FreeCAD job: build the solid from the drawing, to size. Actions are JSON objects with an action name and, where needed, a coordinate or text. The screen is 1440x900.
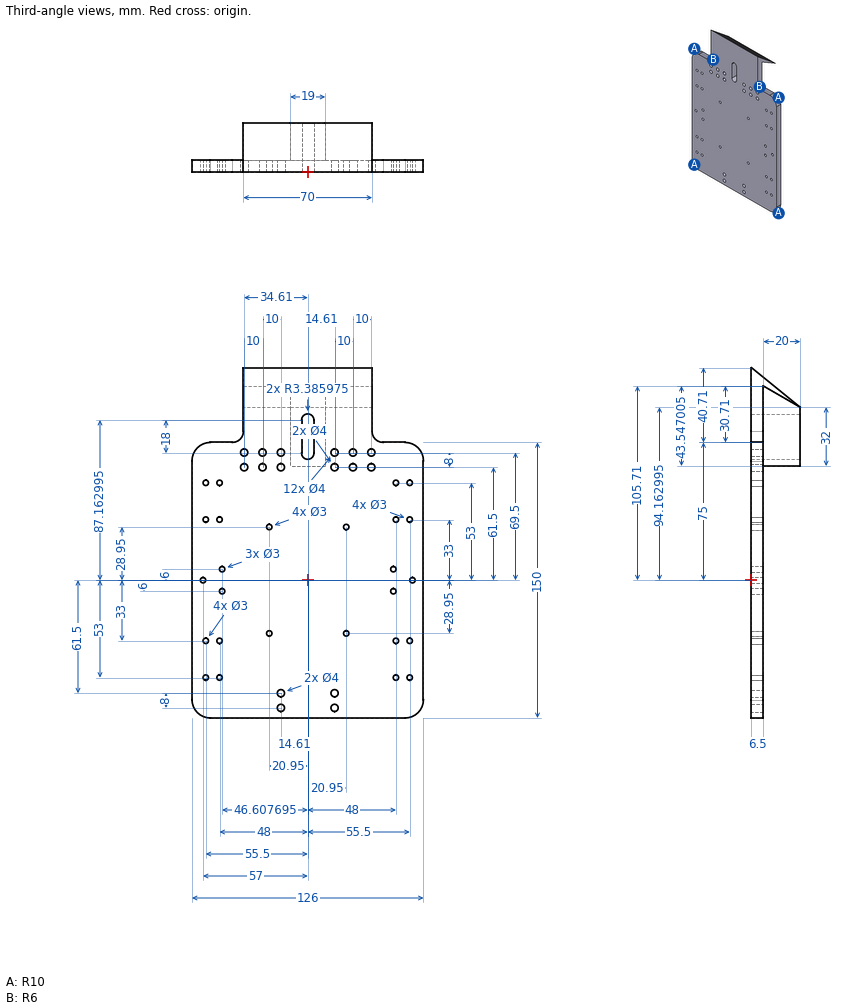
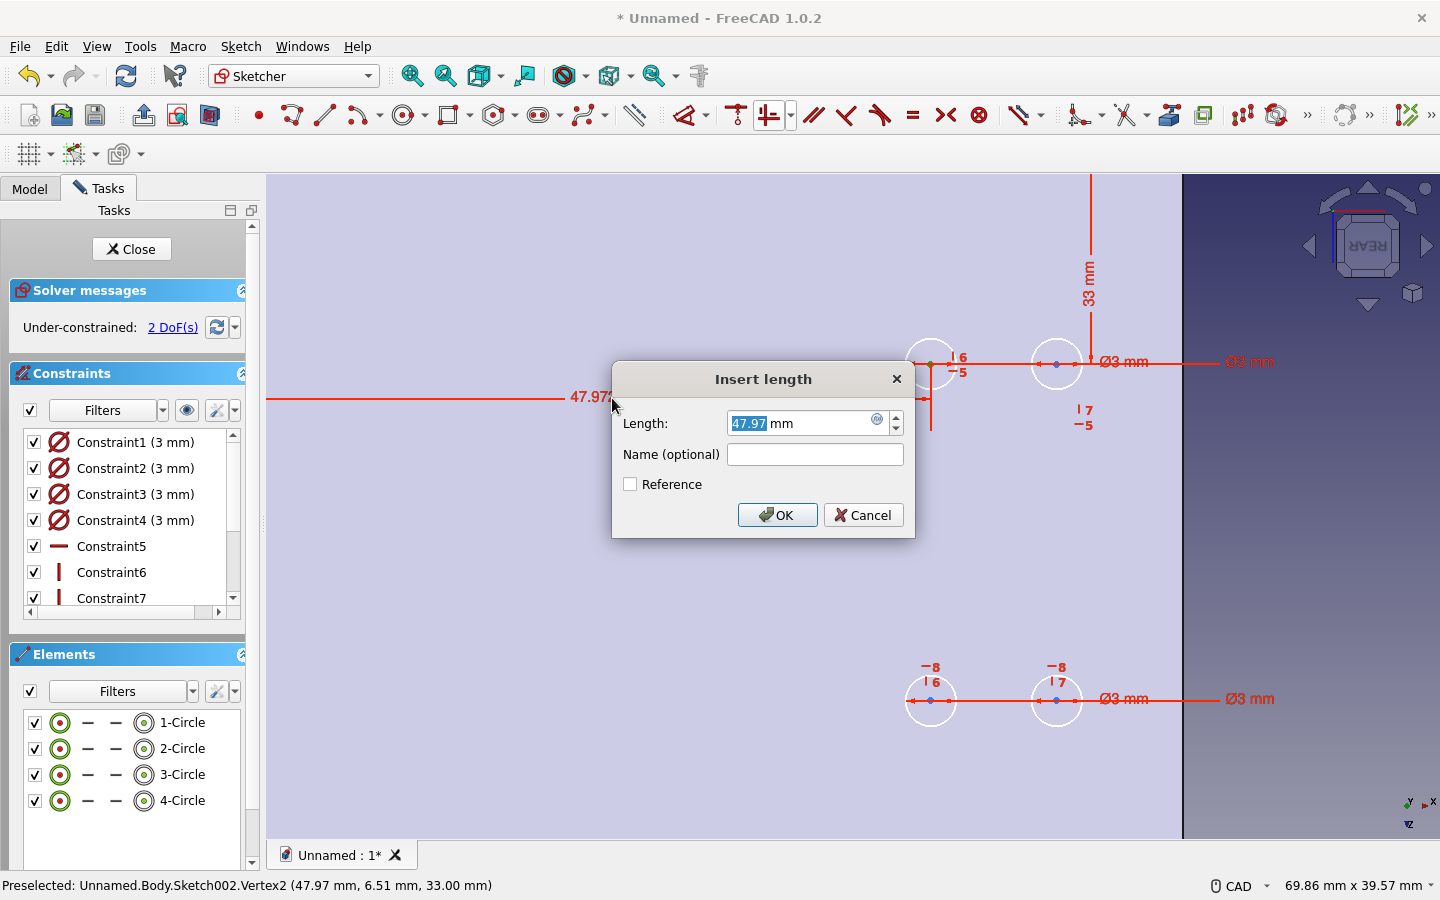
{"action": "type", "text": "48"}
{"action": "key", "text": "Return"}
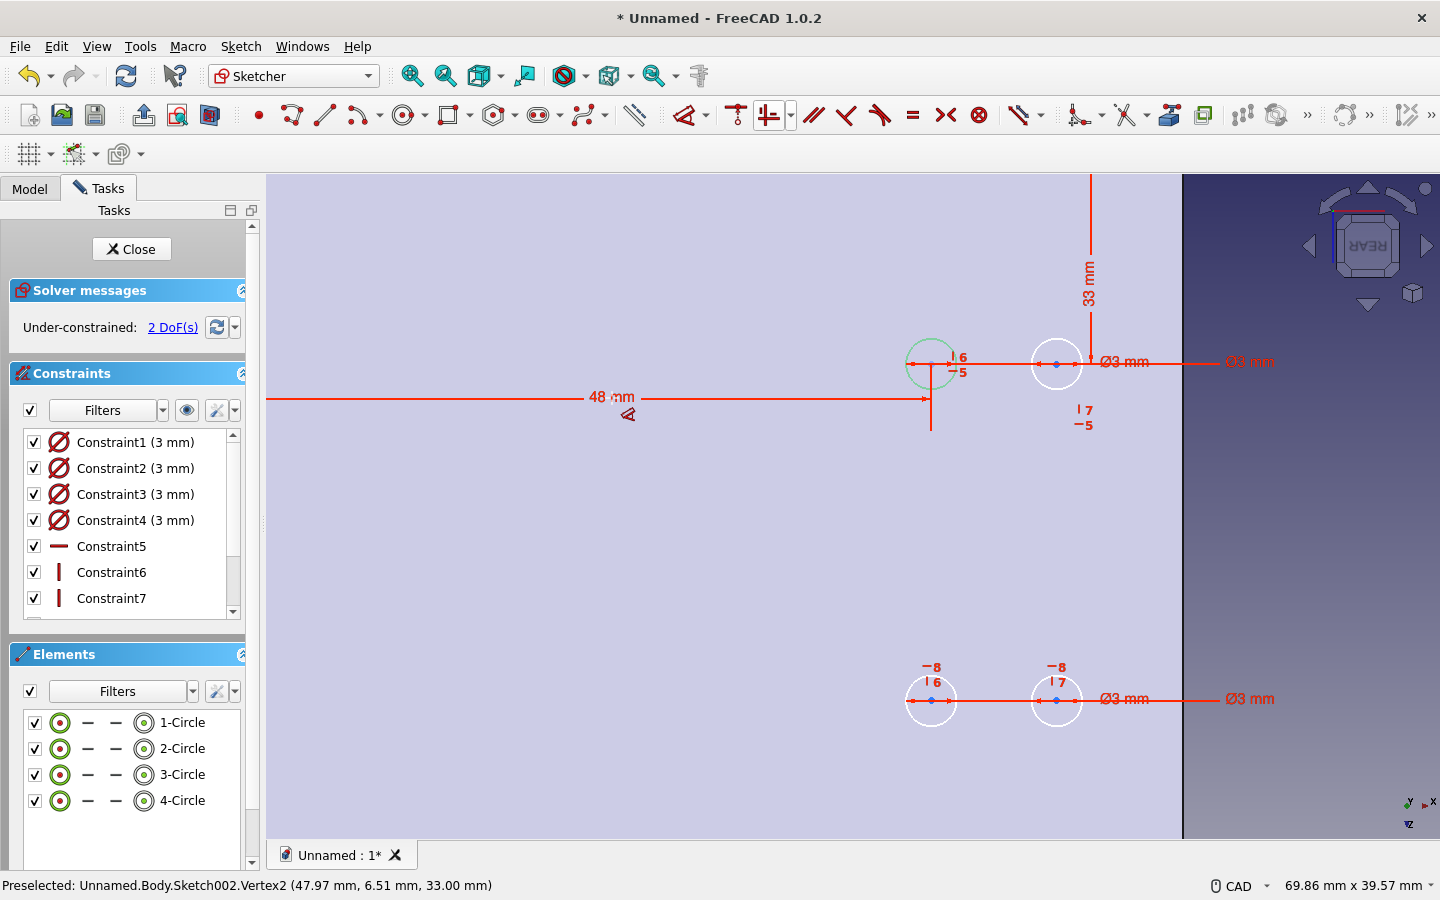
{"action": "left_click", "coordinate": [931, 701]}
{"action": "left_click", "coordinate": [965, 451]}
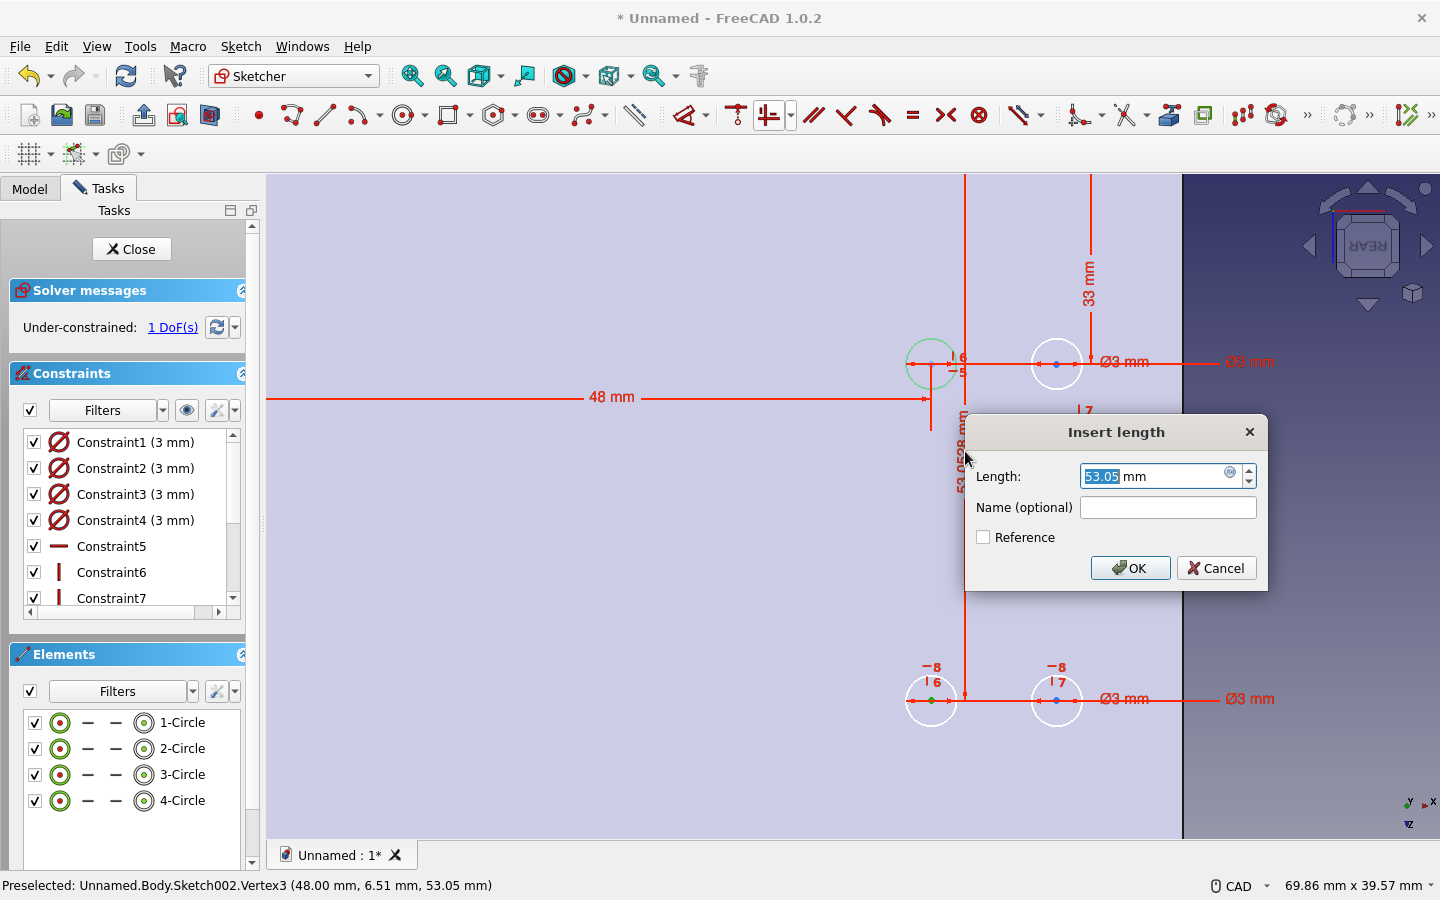
{"action": "type", "text": "53"}
{"action": "key", "text": "Return"}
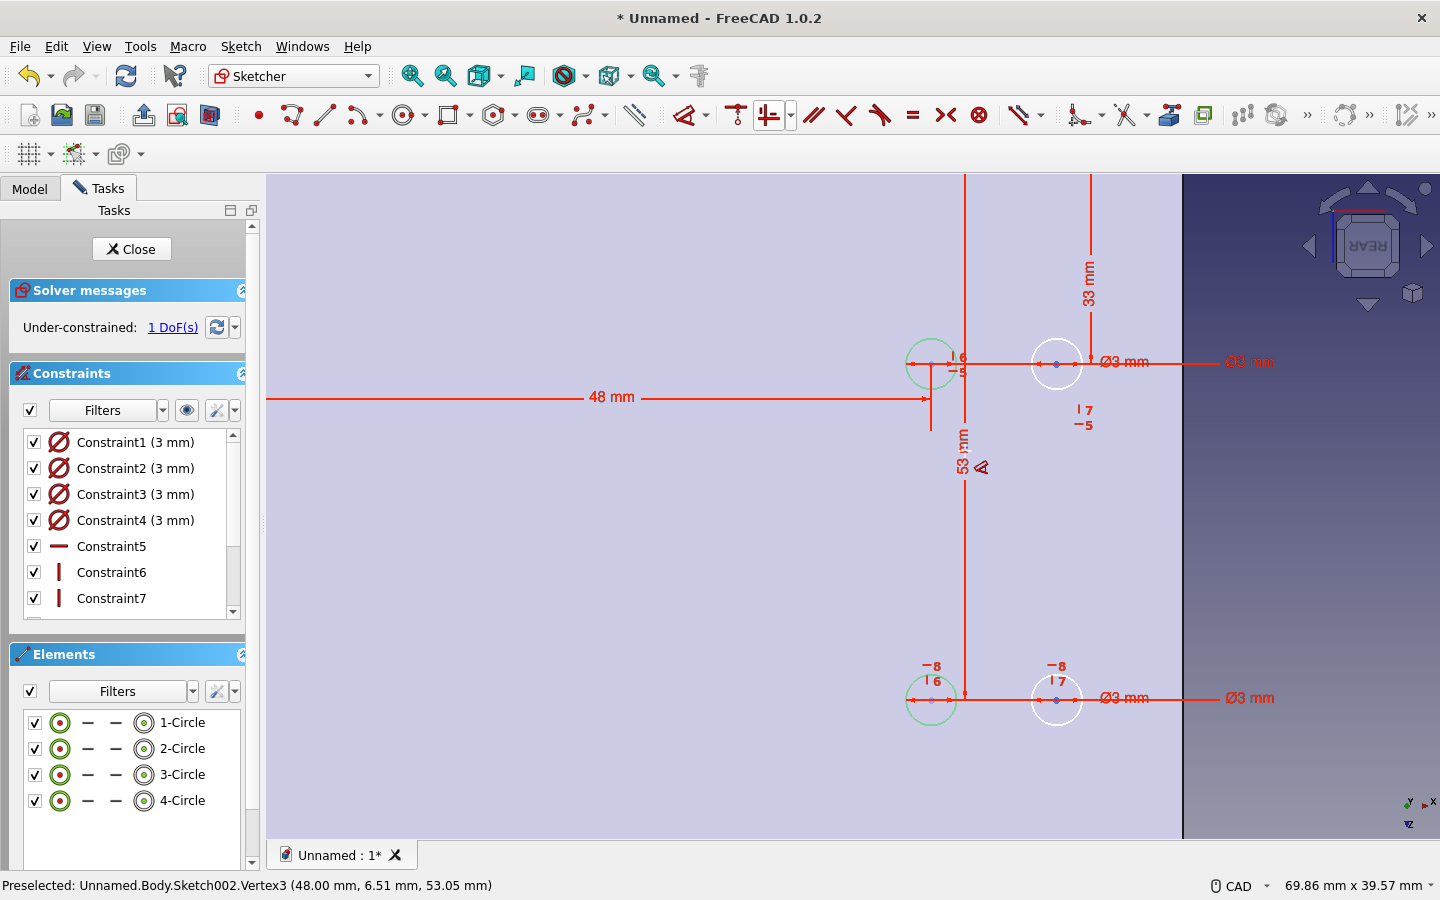
{"action": "left_click", "coordinate": [1057, 364]}
{"action": "left_click", "coordinate": [500, 398]}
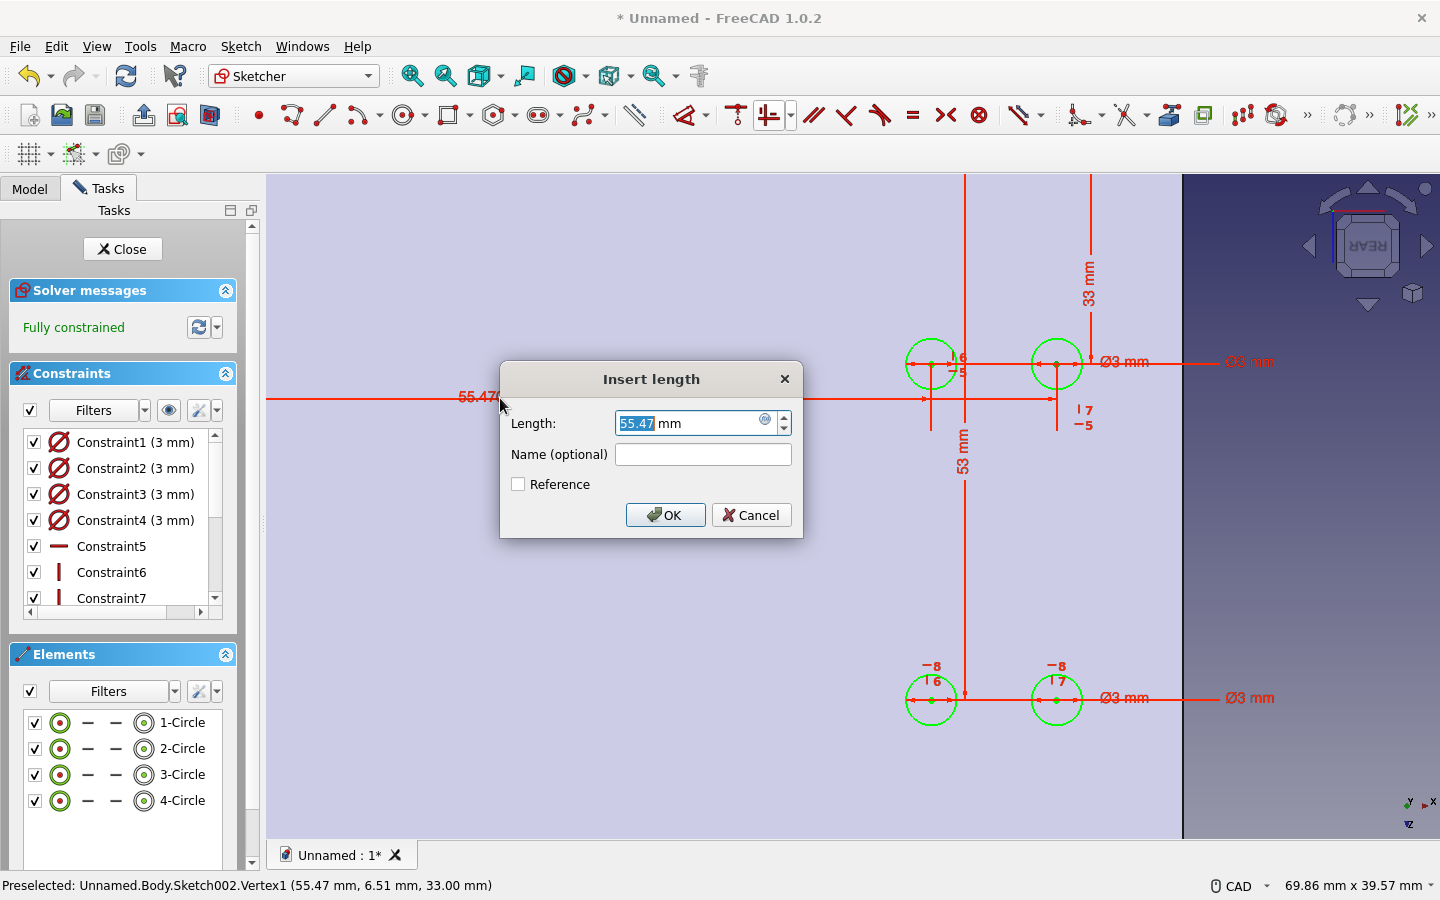
{"action": "type", "text": "55.5"}
{"action": "key", "text": "Return"}
{"action": "key", "text": "Escape"}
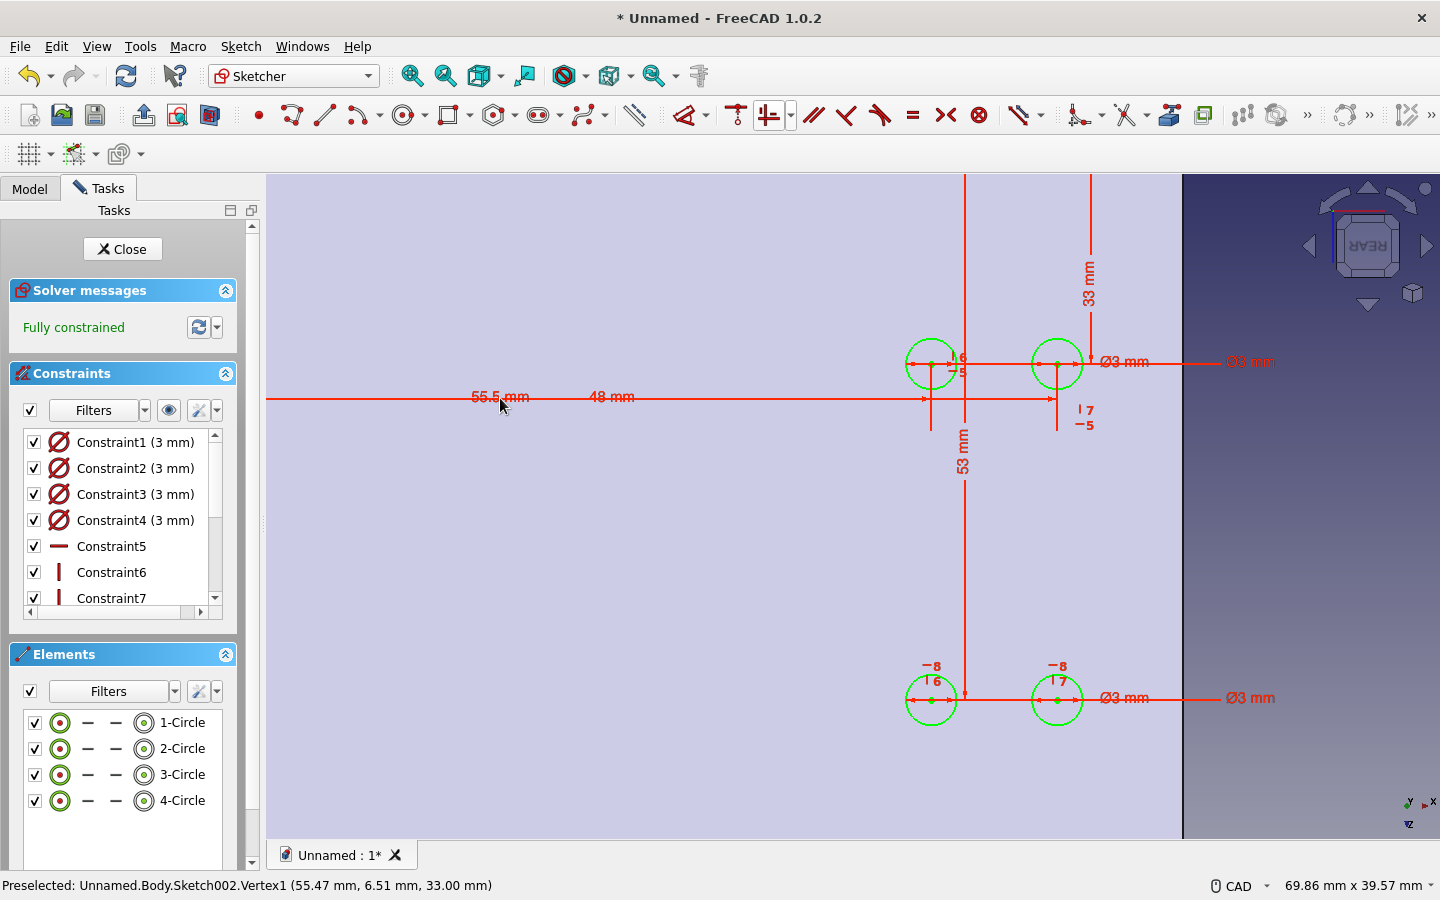
{"action": "left_click", "coordinate": [123, 249]}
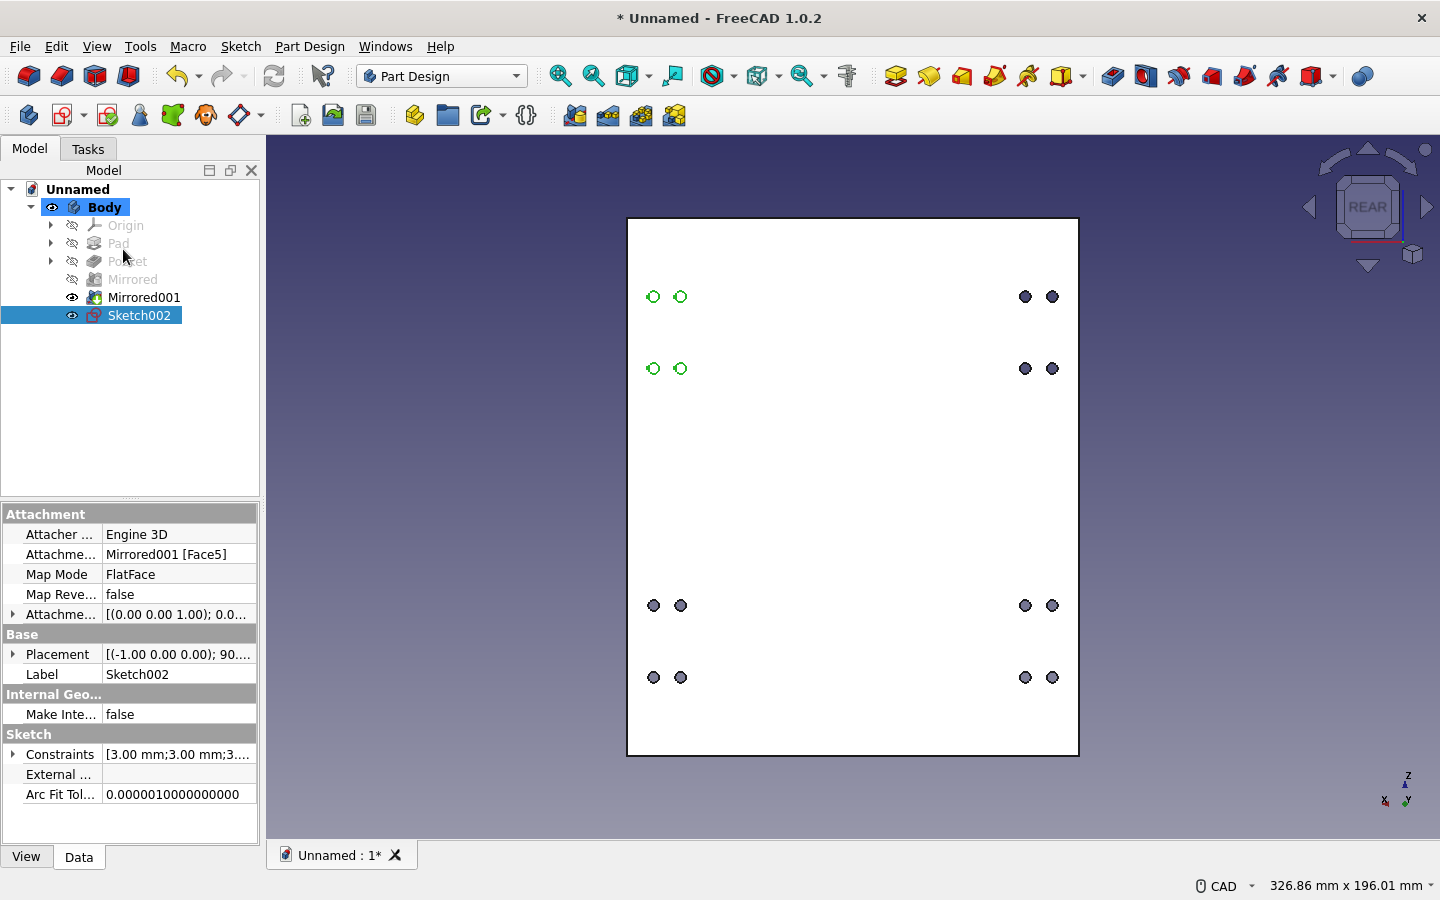
{"action": "left_click", "coordinate": [1113, 76]}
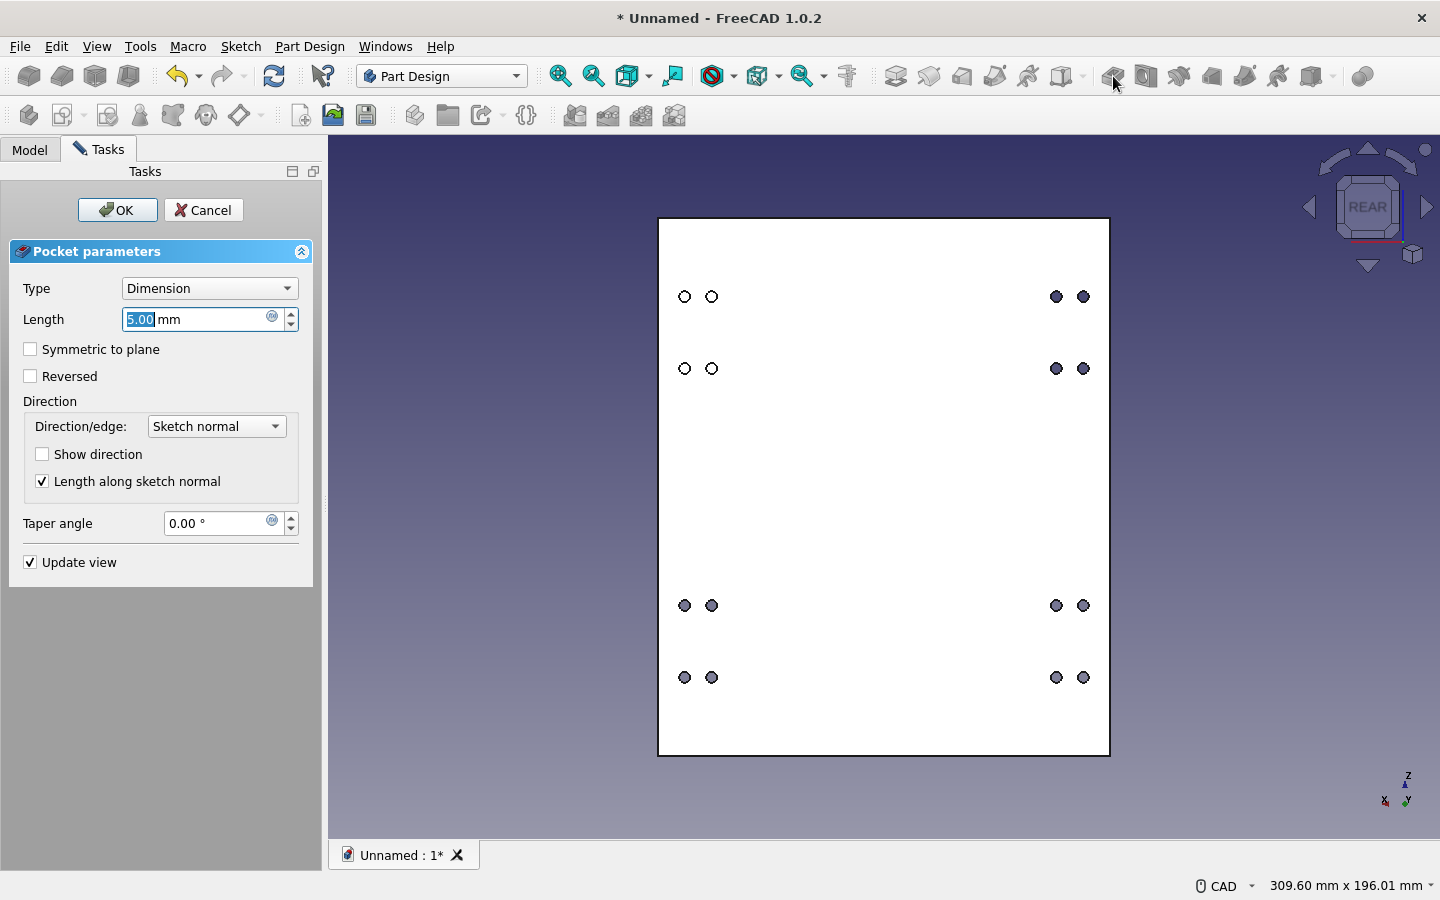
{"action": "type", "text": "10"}
{"action": "key", "text": "Tab"}